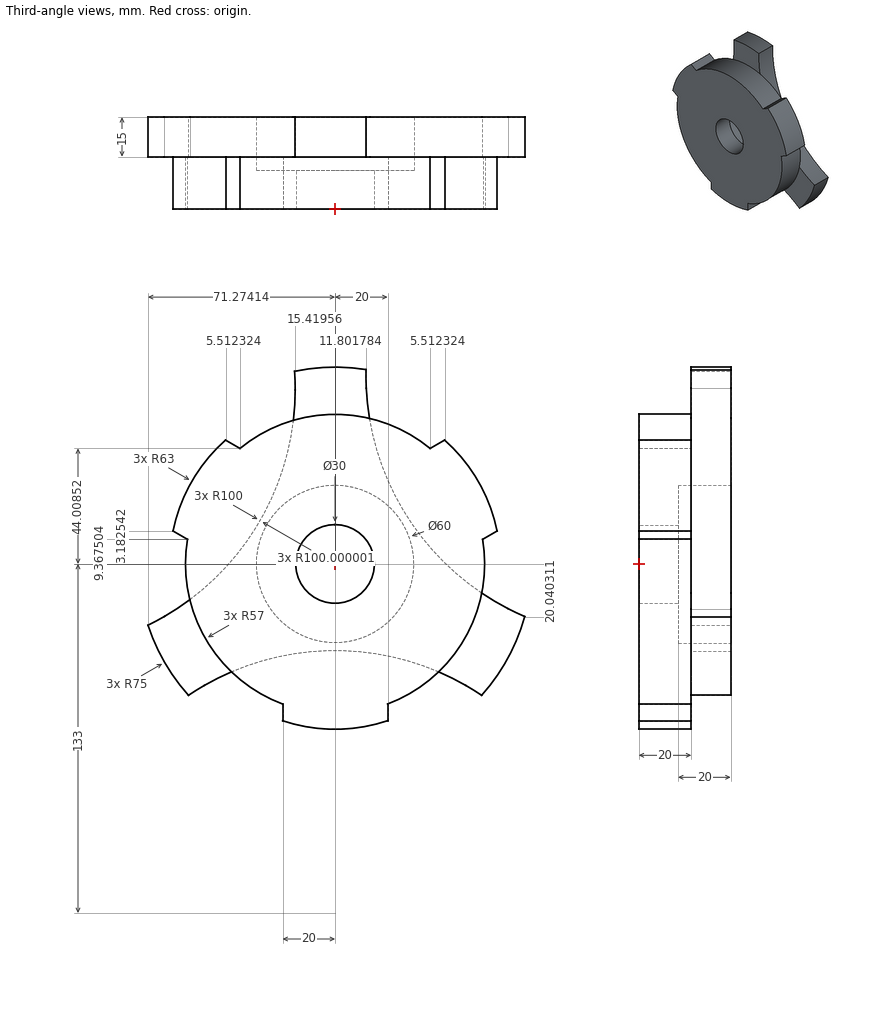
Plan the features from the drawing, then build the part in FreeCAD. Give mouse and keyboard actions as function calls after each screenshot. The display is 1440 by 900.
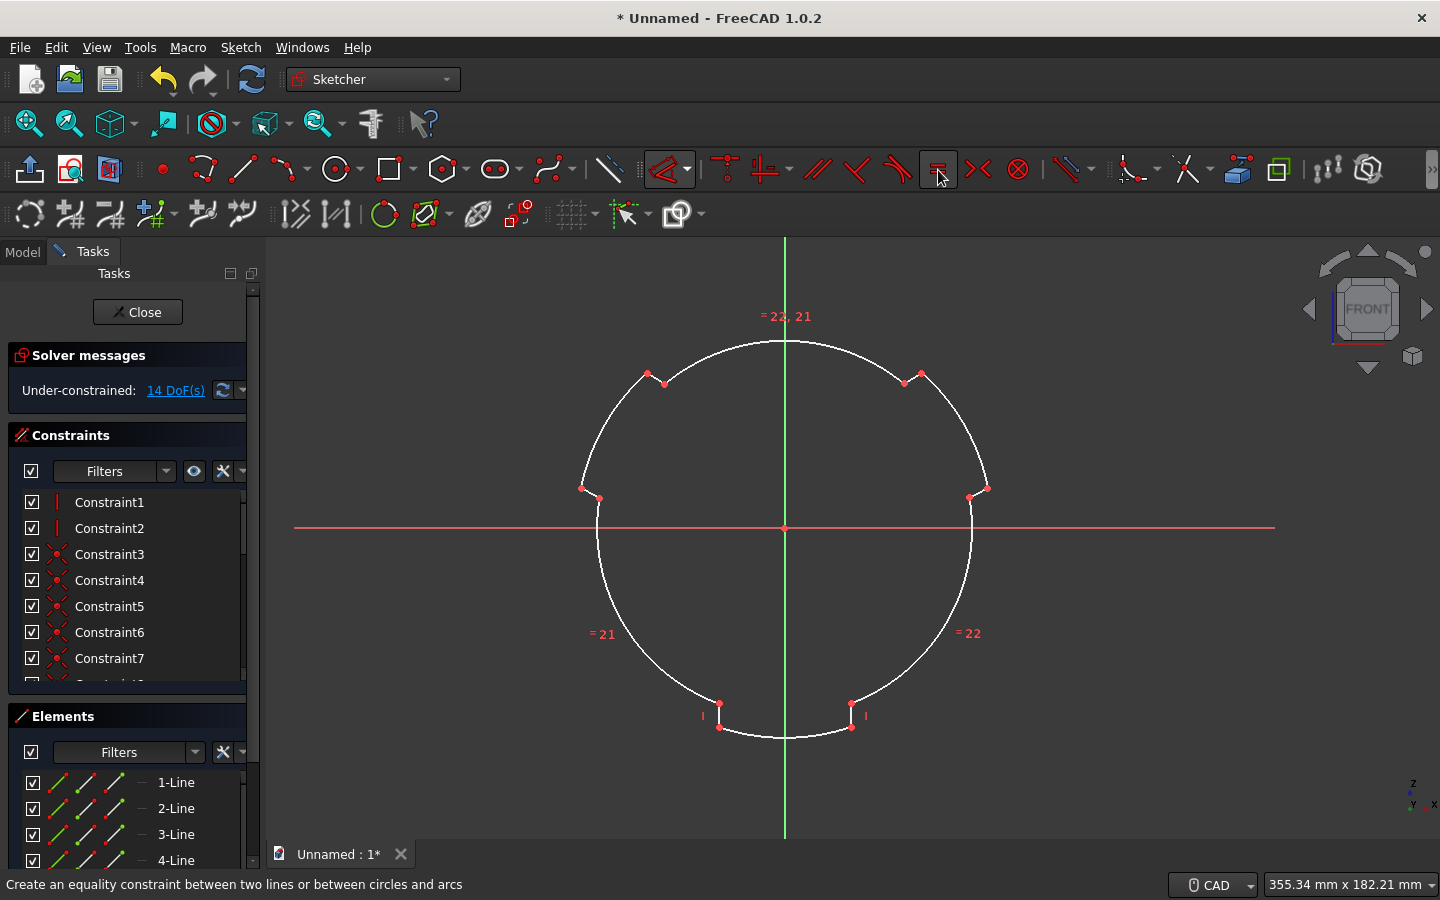
click(620, 403)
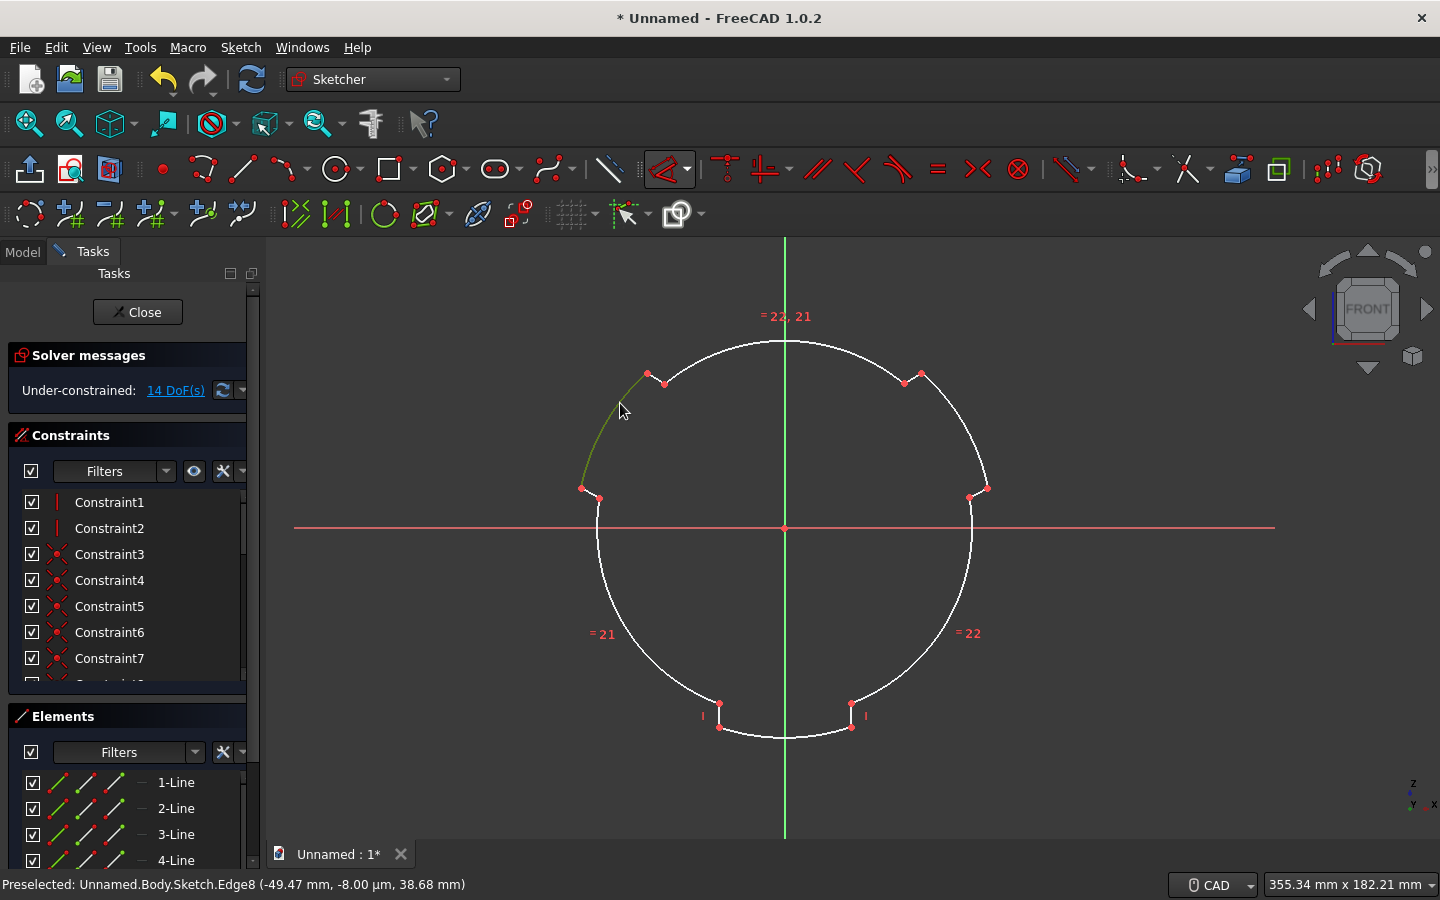
click(976, 449)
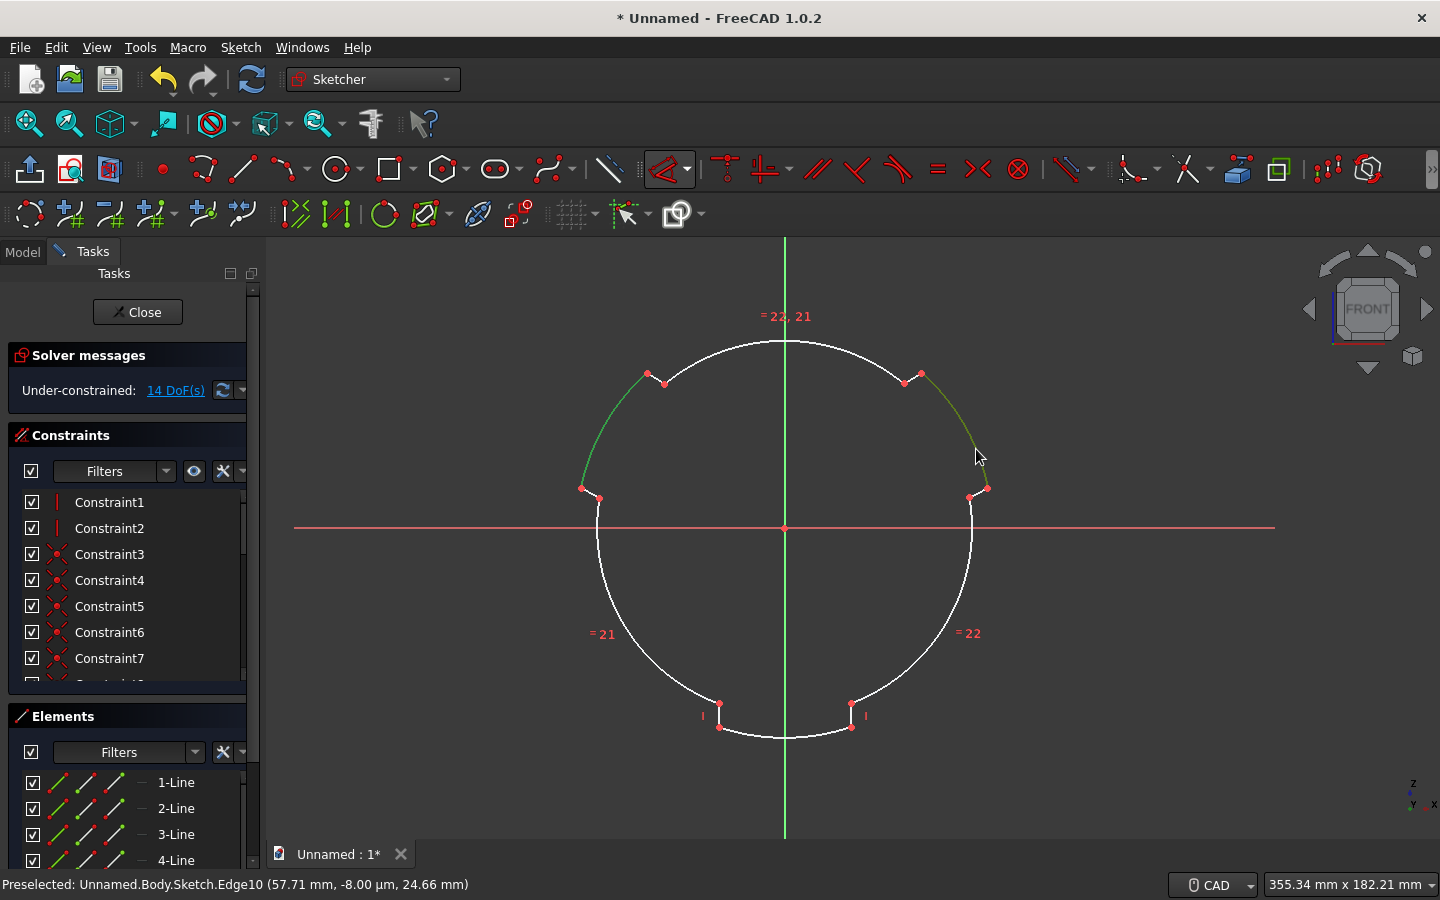
click(758, 736)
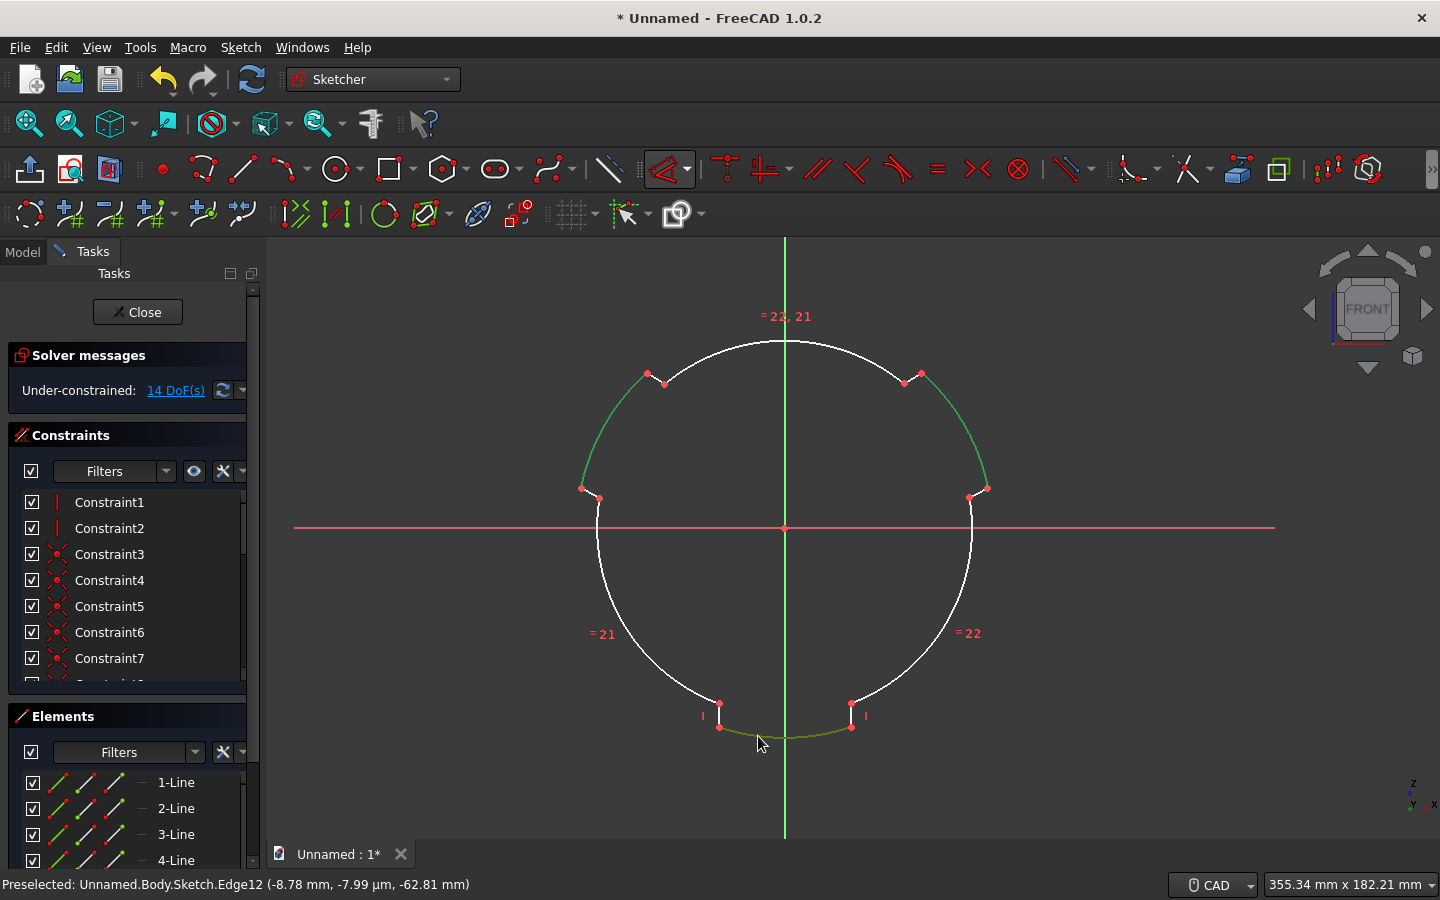
key(e)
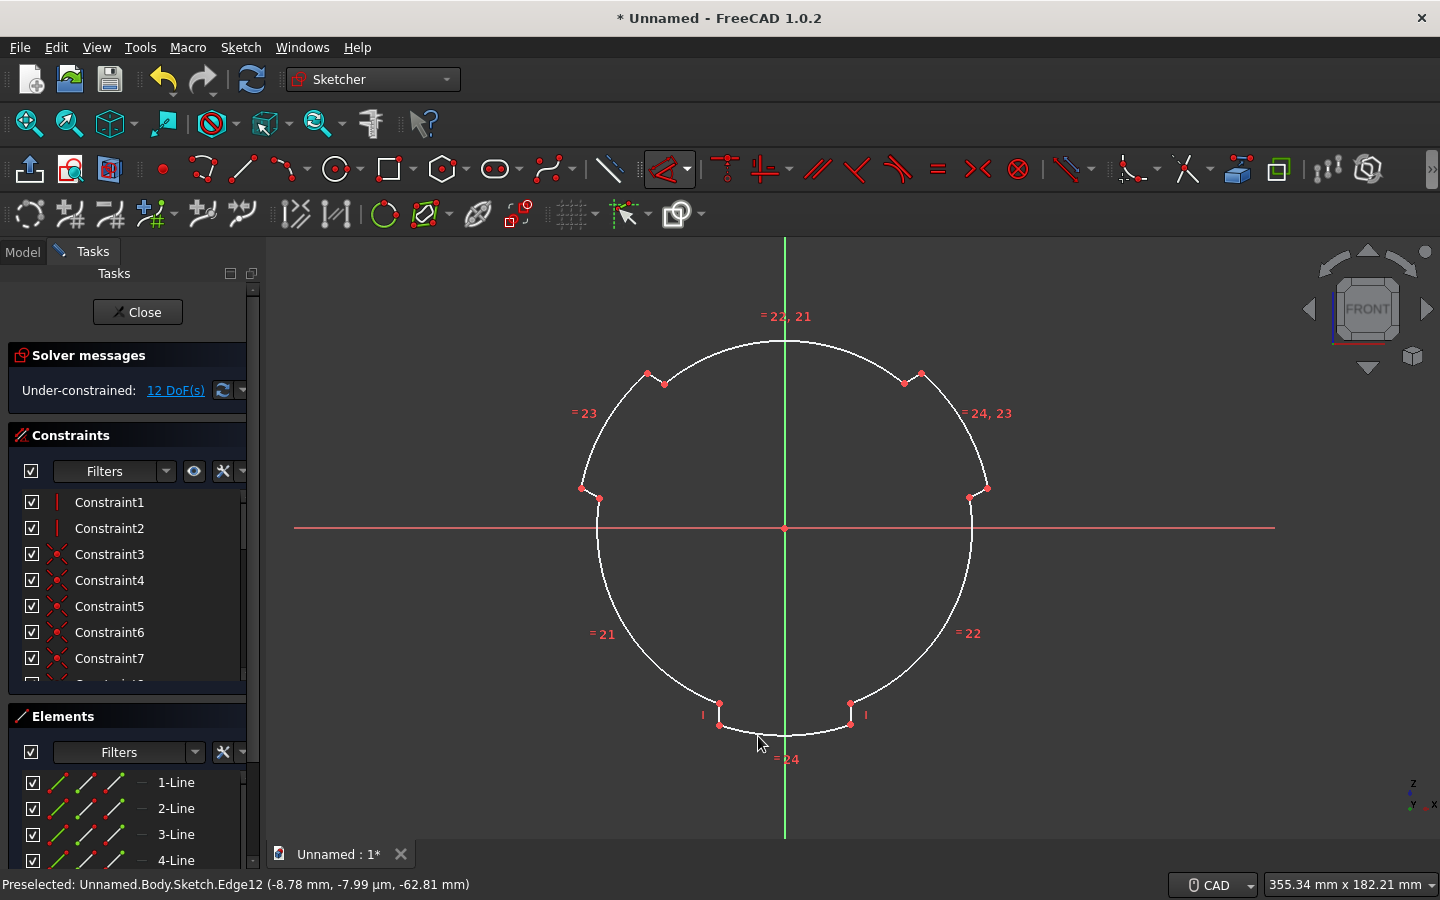
click(664, 170)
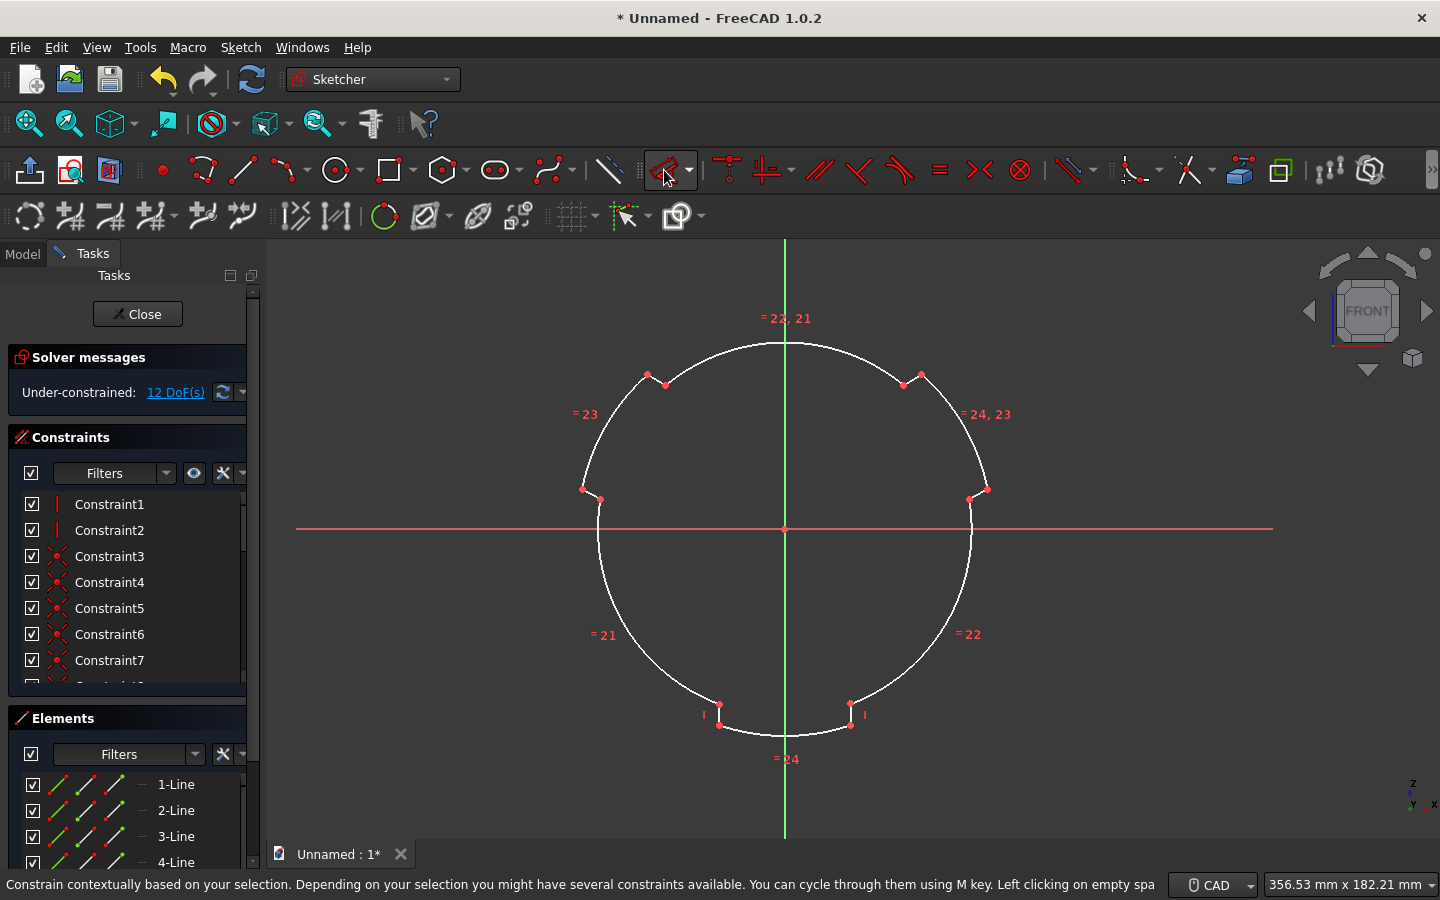
click(604, 576)
click(573, 584)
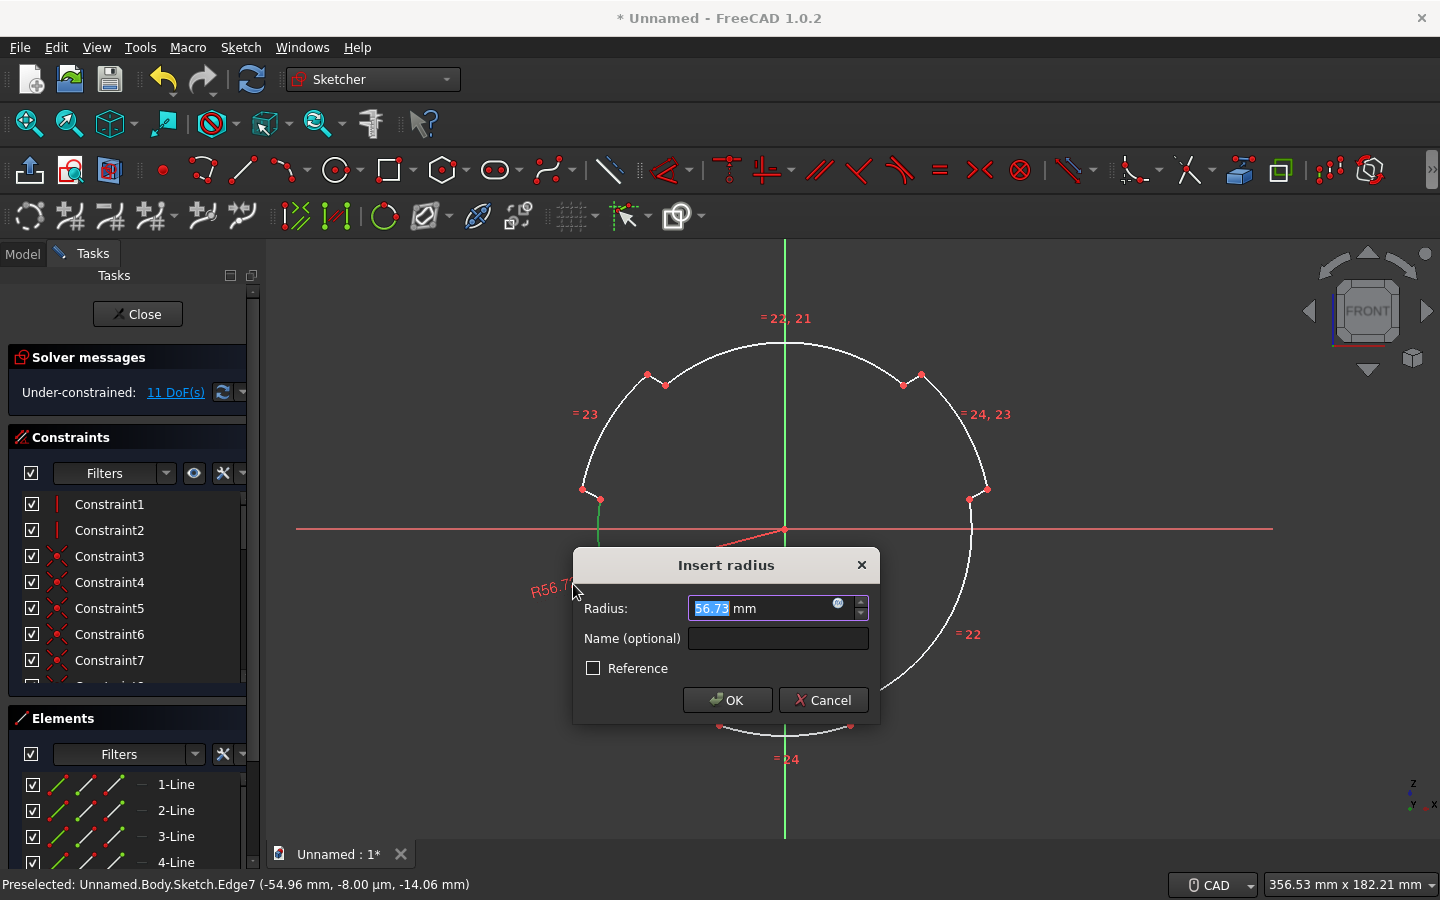
text(57)
key(Return)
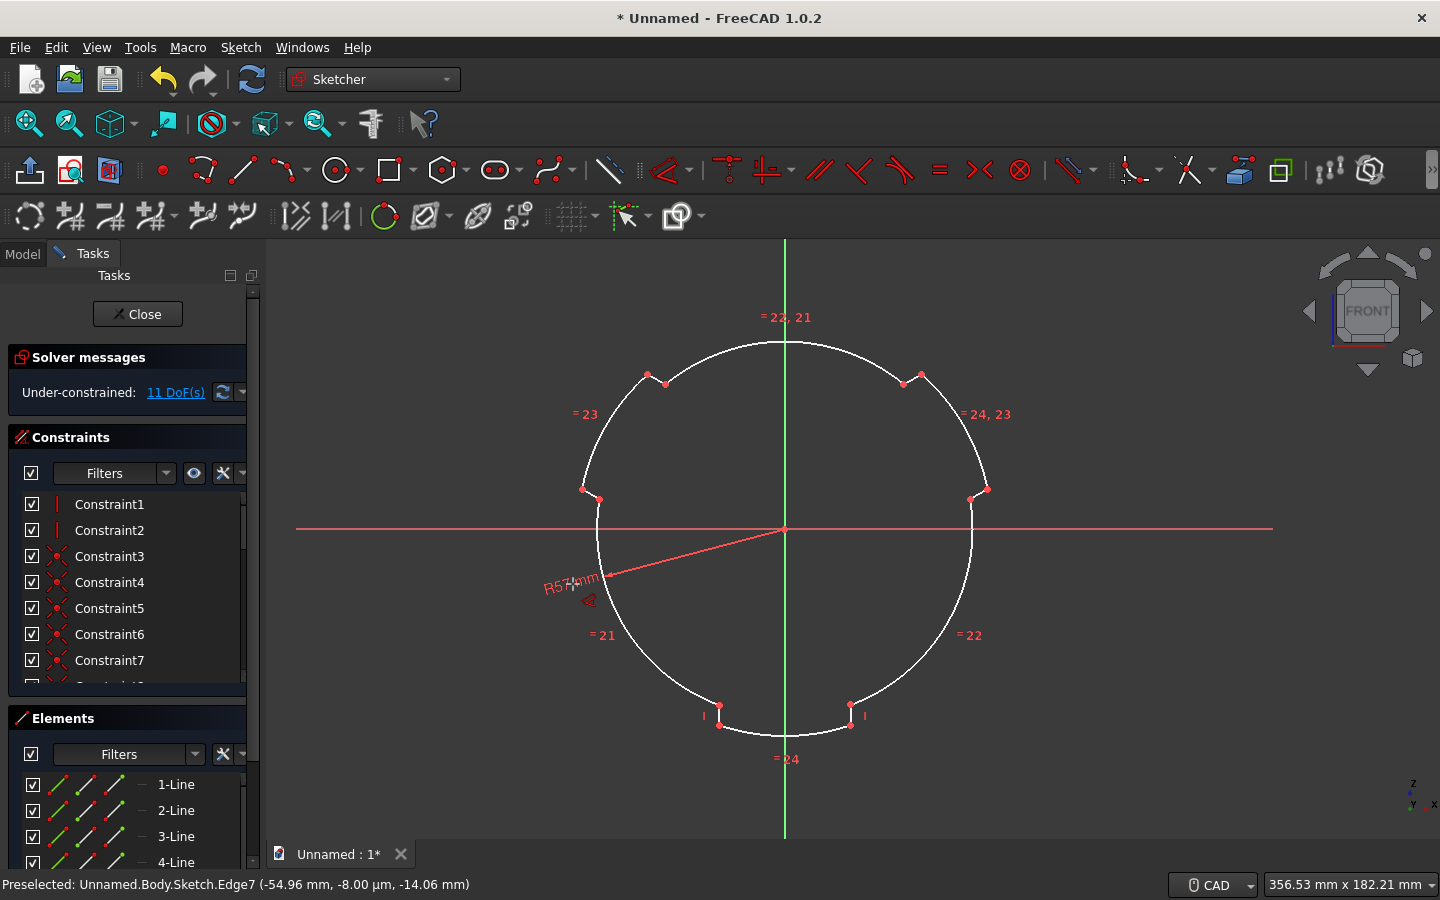
click(620, 404)
click(595, 385)